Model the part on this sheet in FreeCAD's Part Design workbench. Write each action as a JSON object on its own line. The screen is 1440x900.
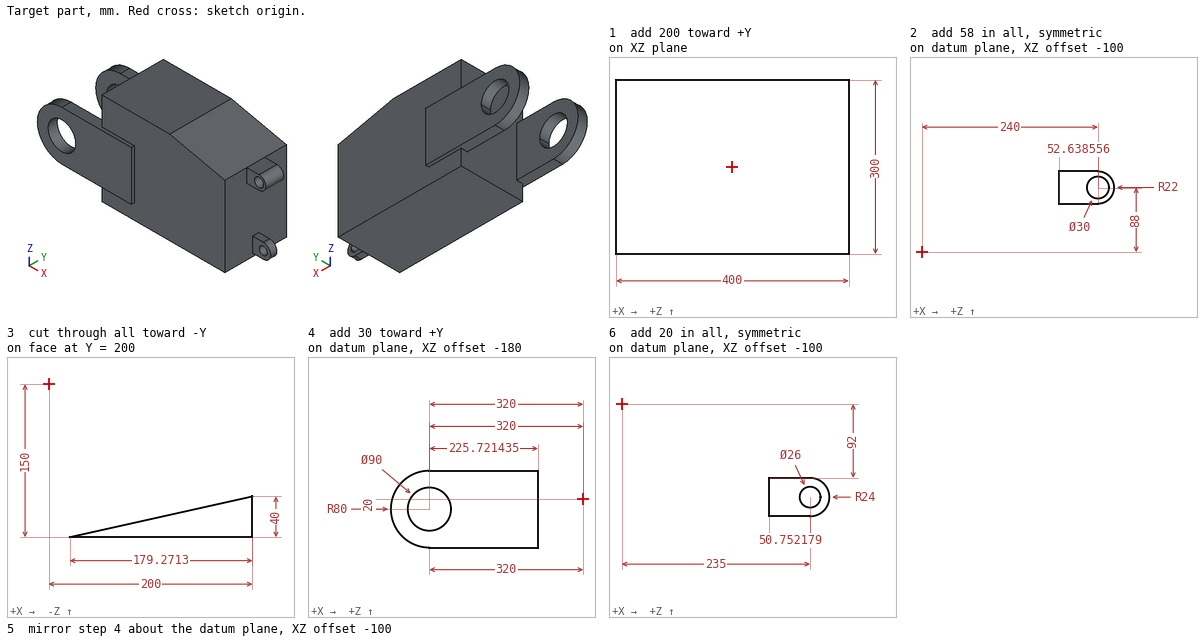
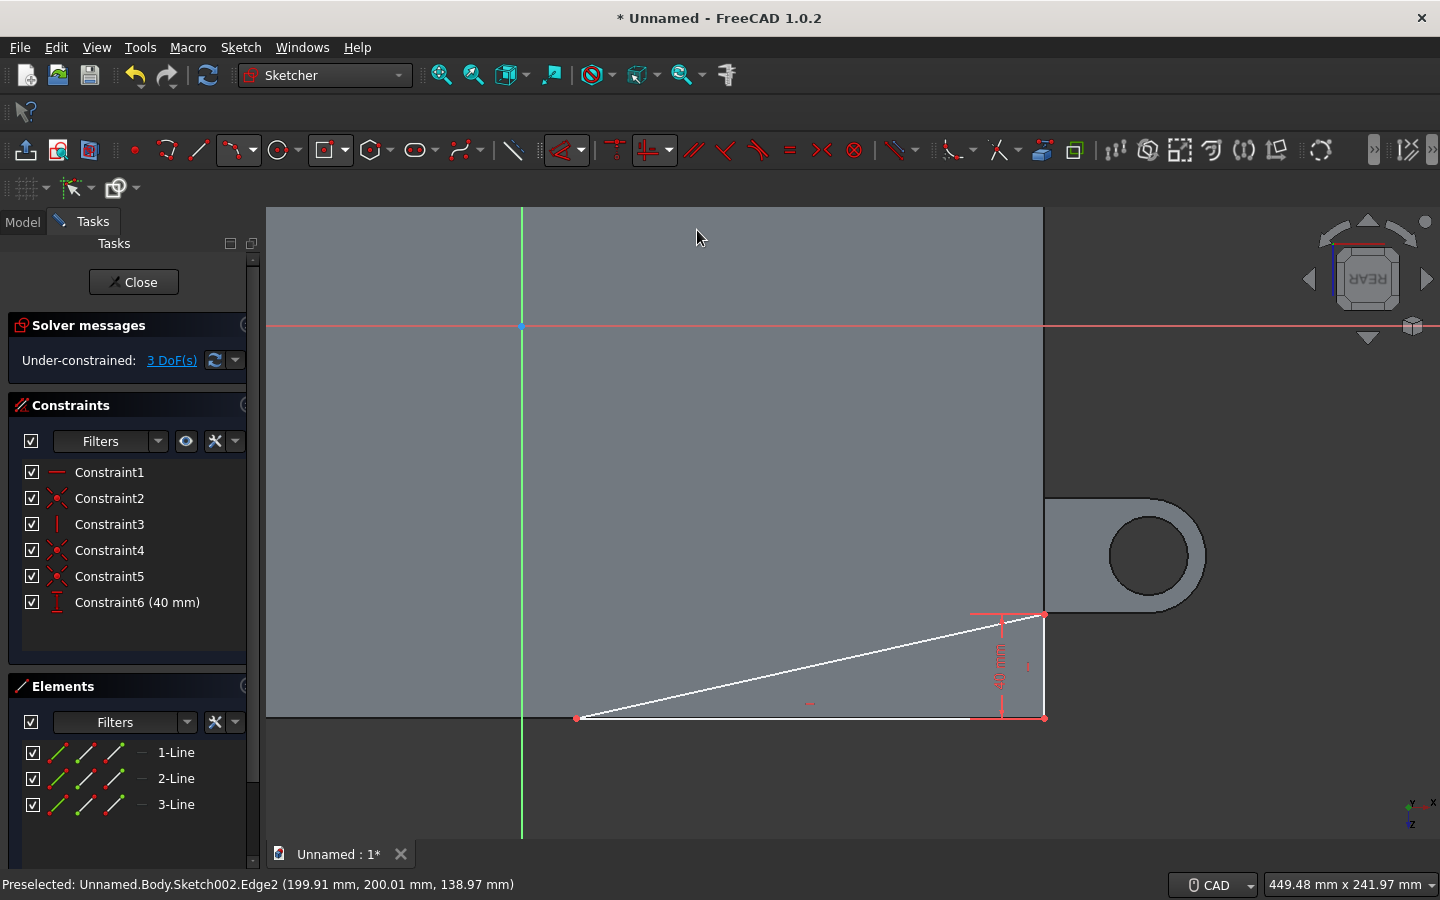
{"action": "left_click", "coordinate": [576, 719]}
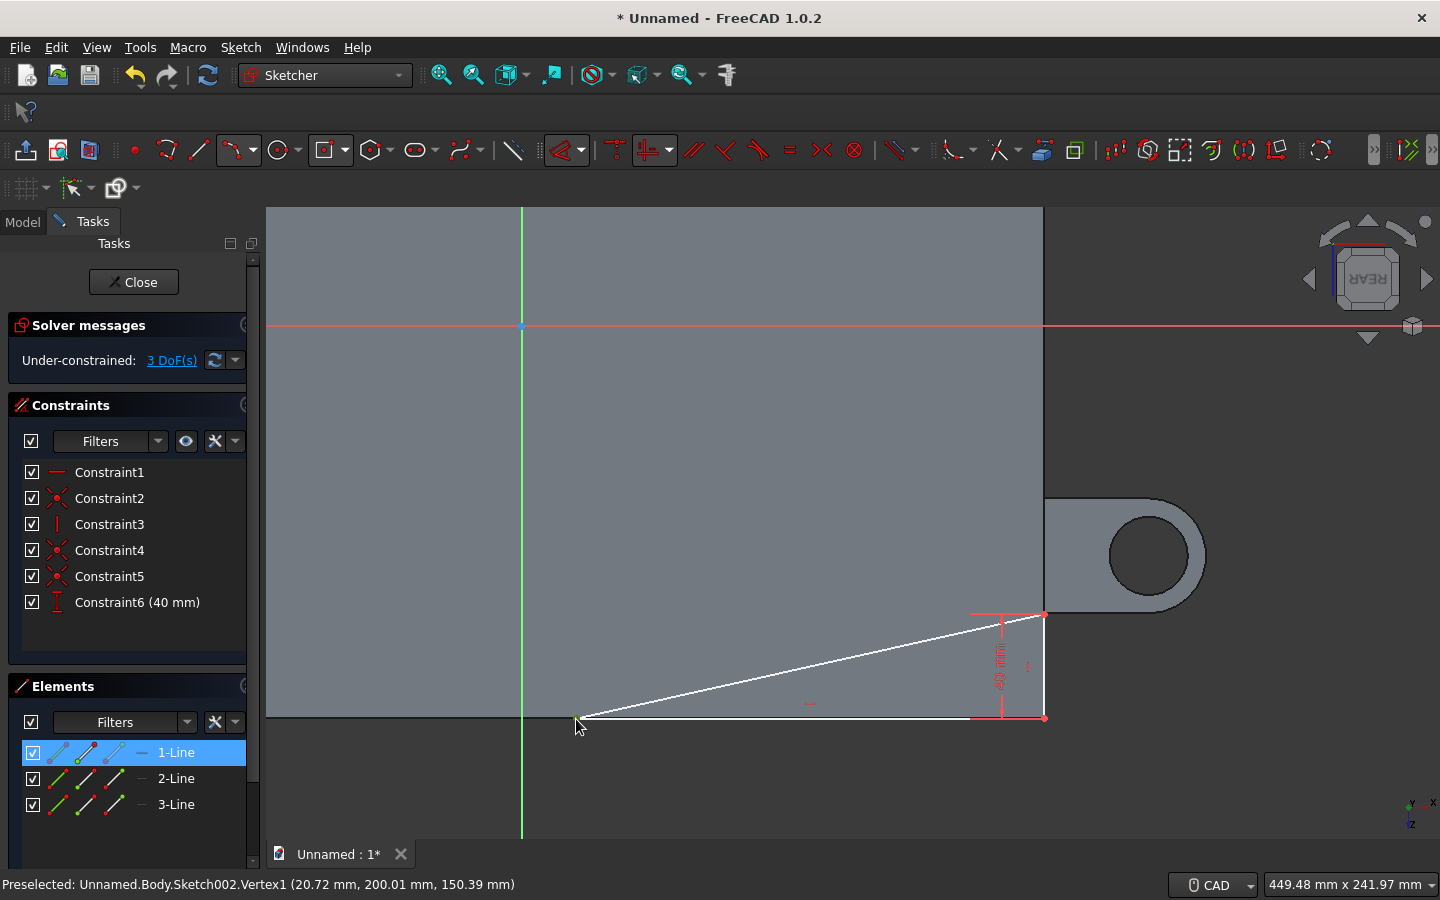
{"action": "left_click", "coordinate": [584, 150]}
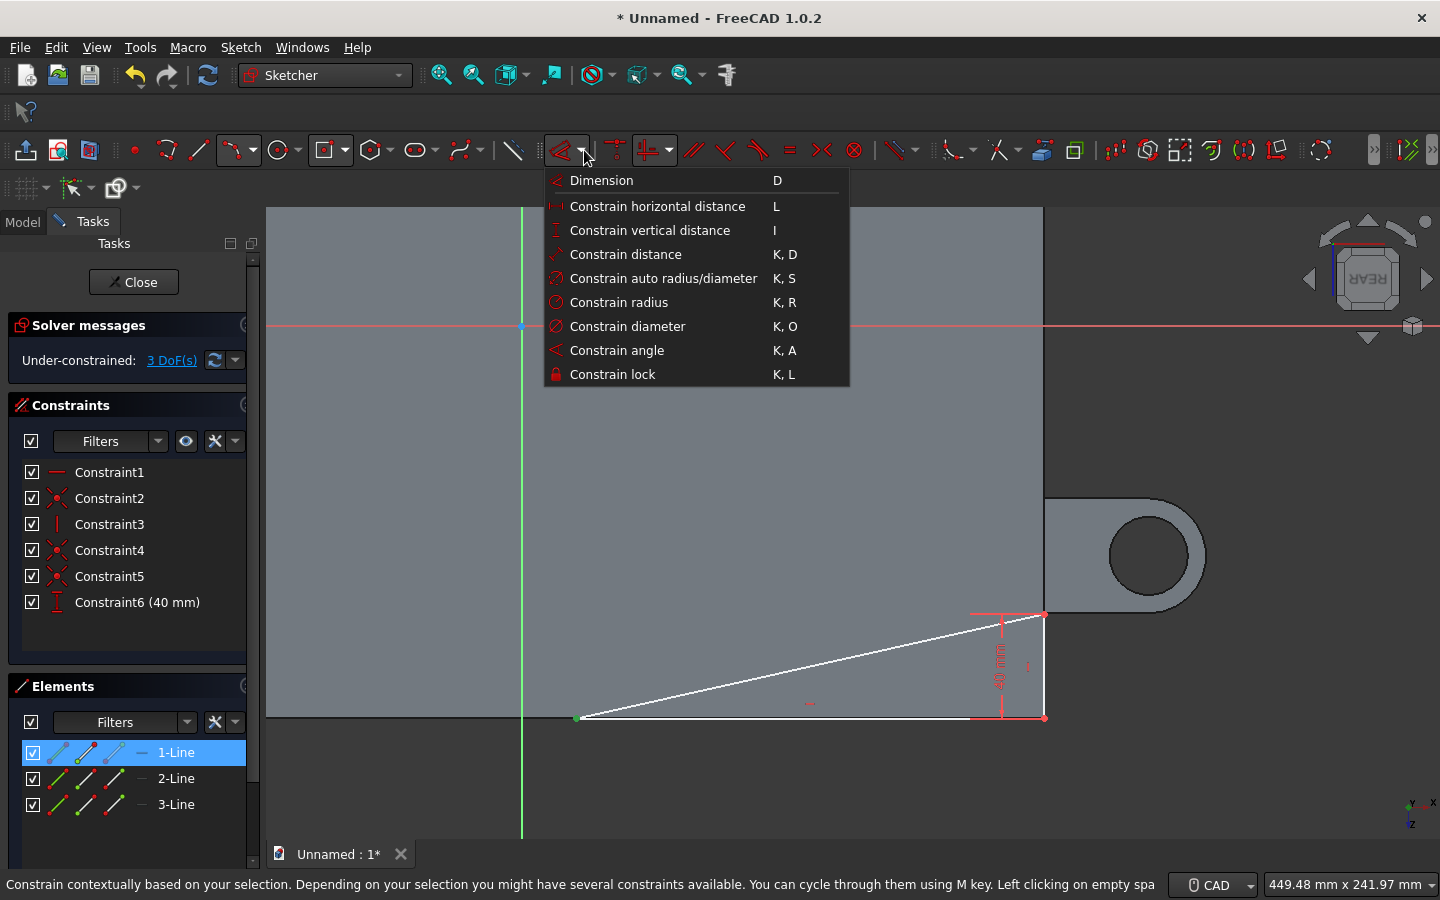
{"action": "left_click", "coordinate": [697, 230]}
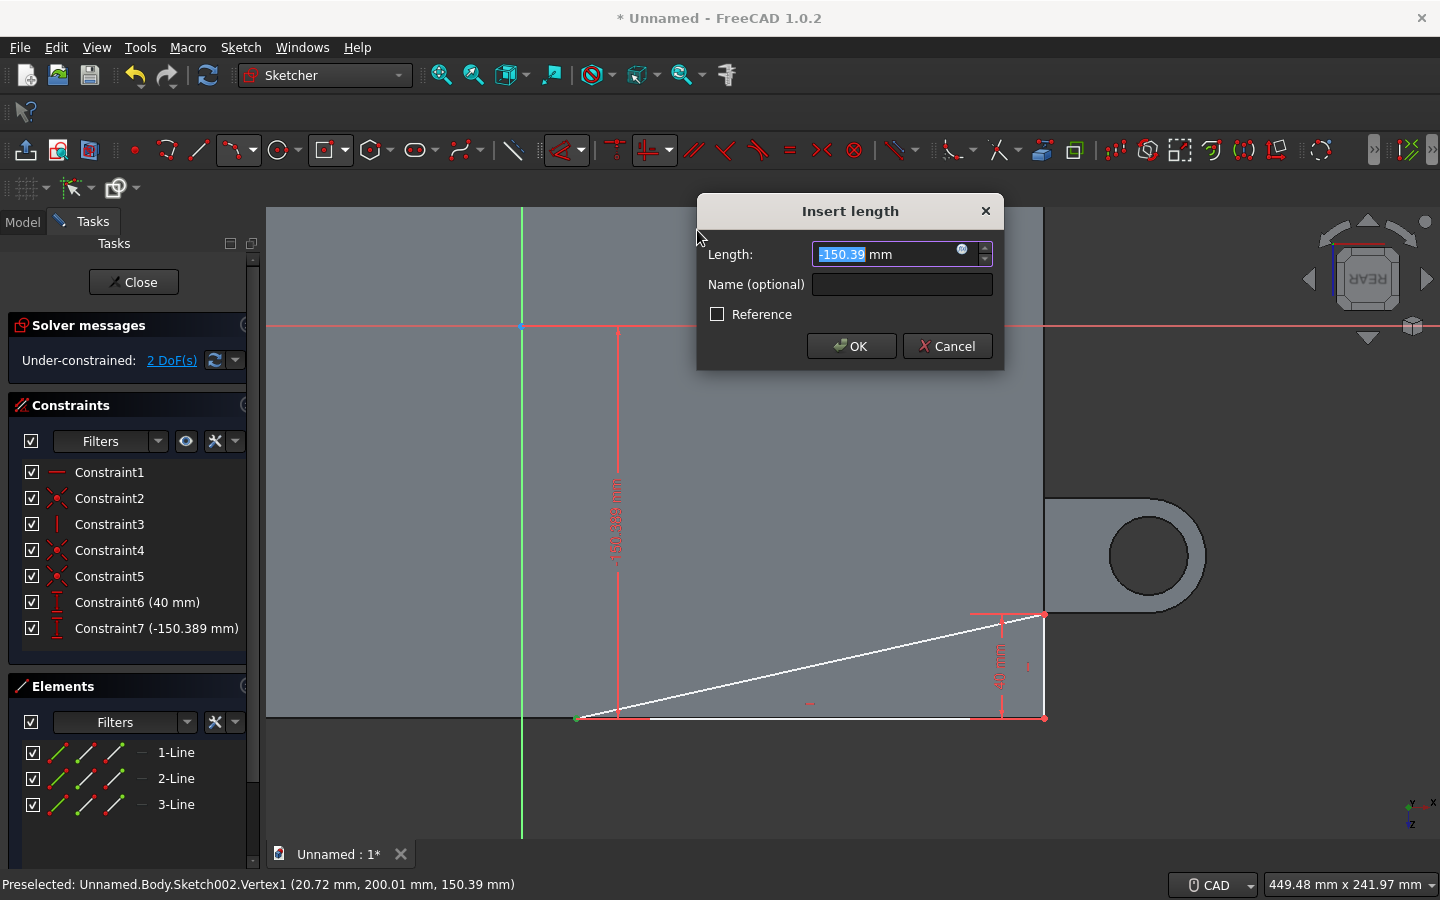
{"action": "type", "text": "-150"}
{"action": "key", "text": "Return"}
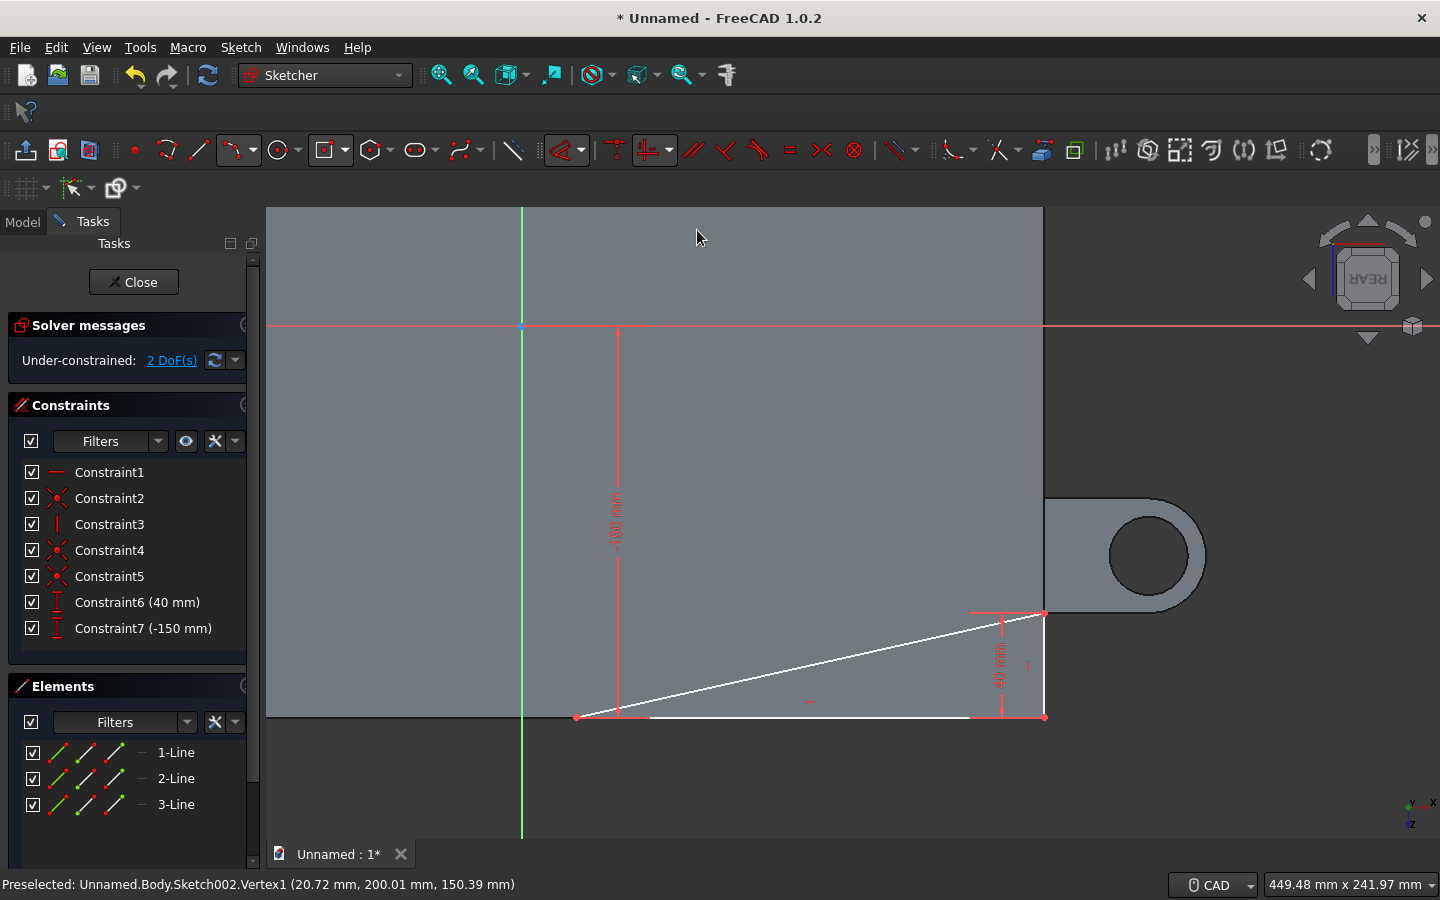
{"action": "left_click", "coordinate": [1044, 718]}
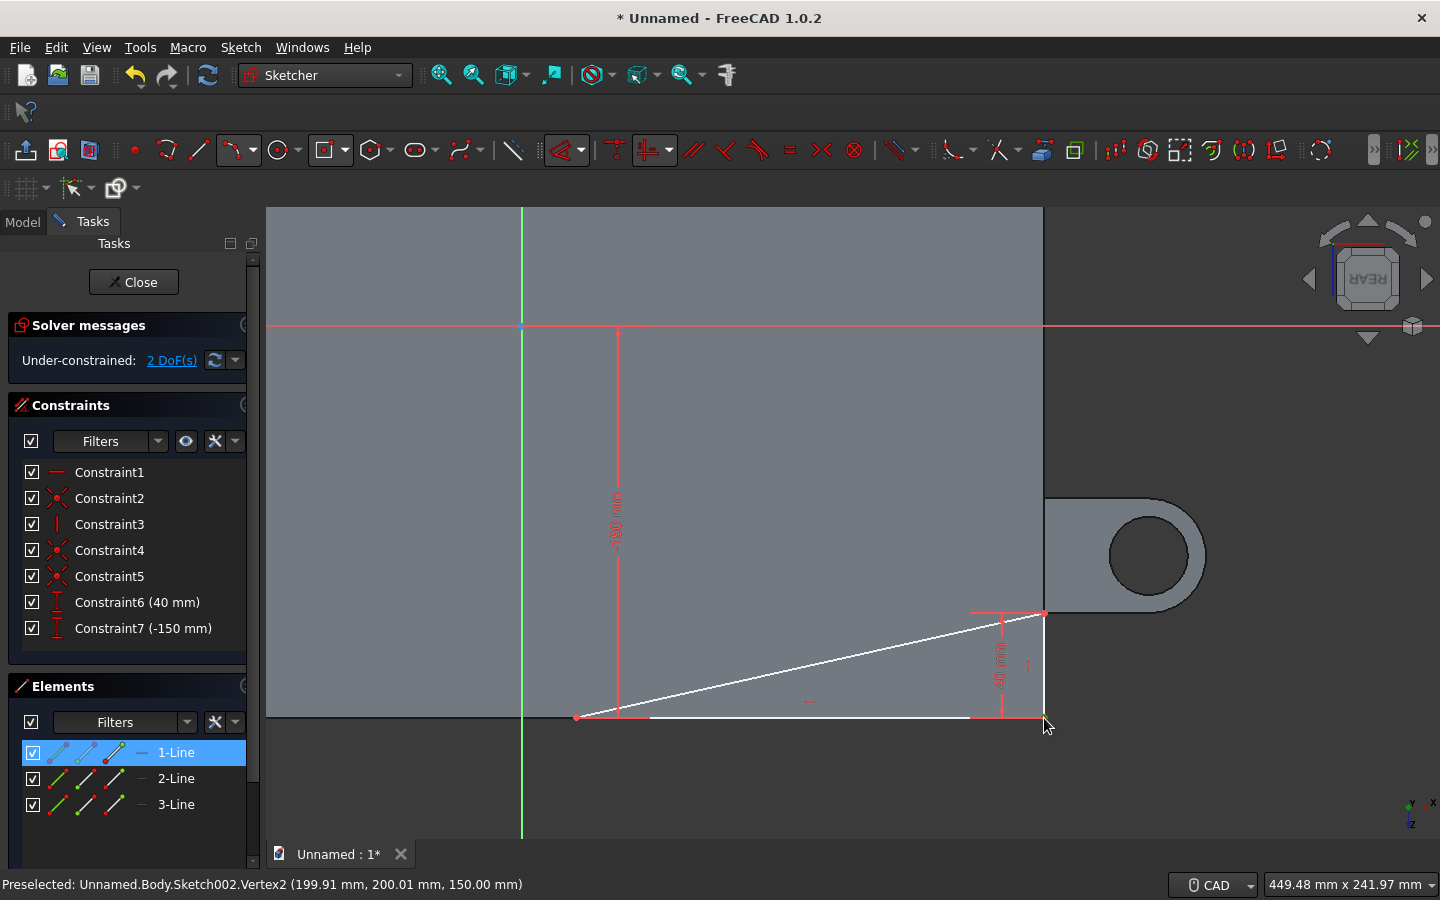
{"action": "left_click", "coordinate": [584, 150]}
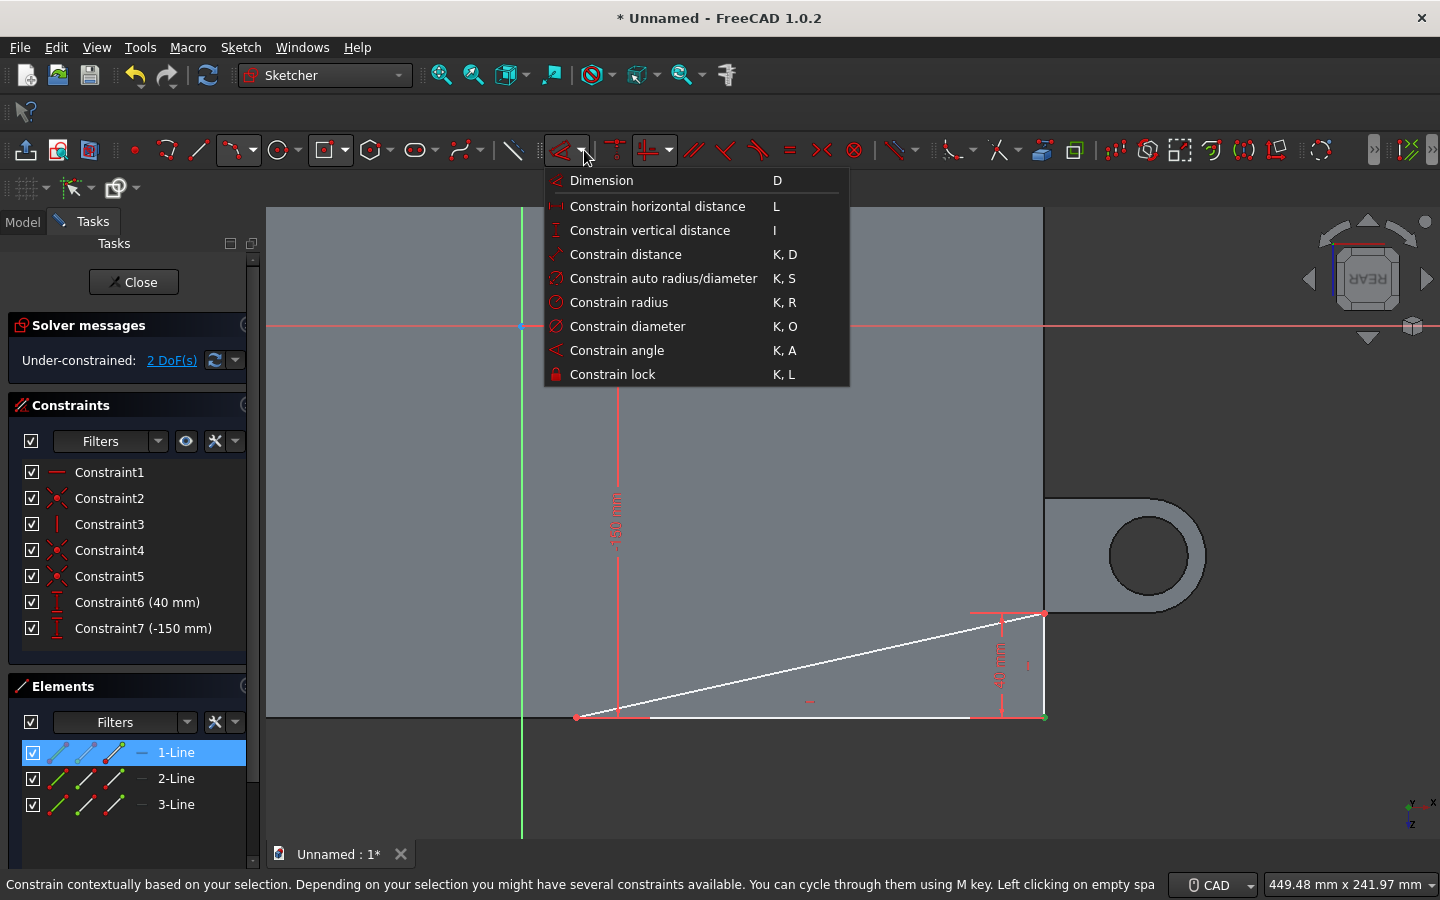
{"action": "left_click", "coordinate": [697, 206]}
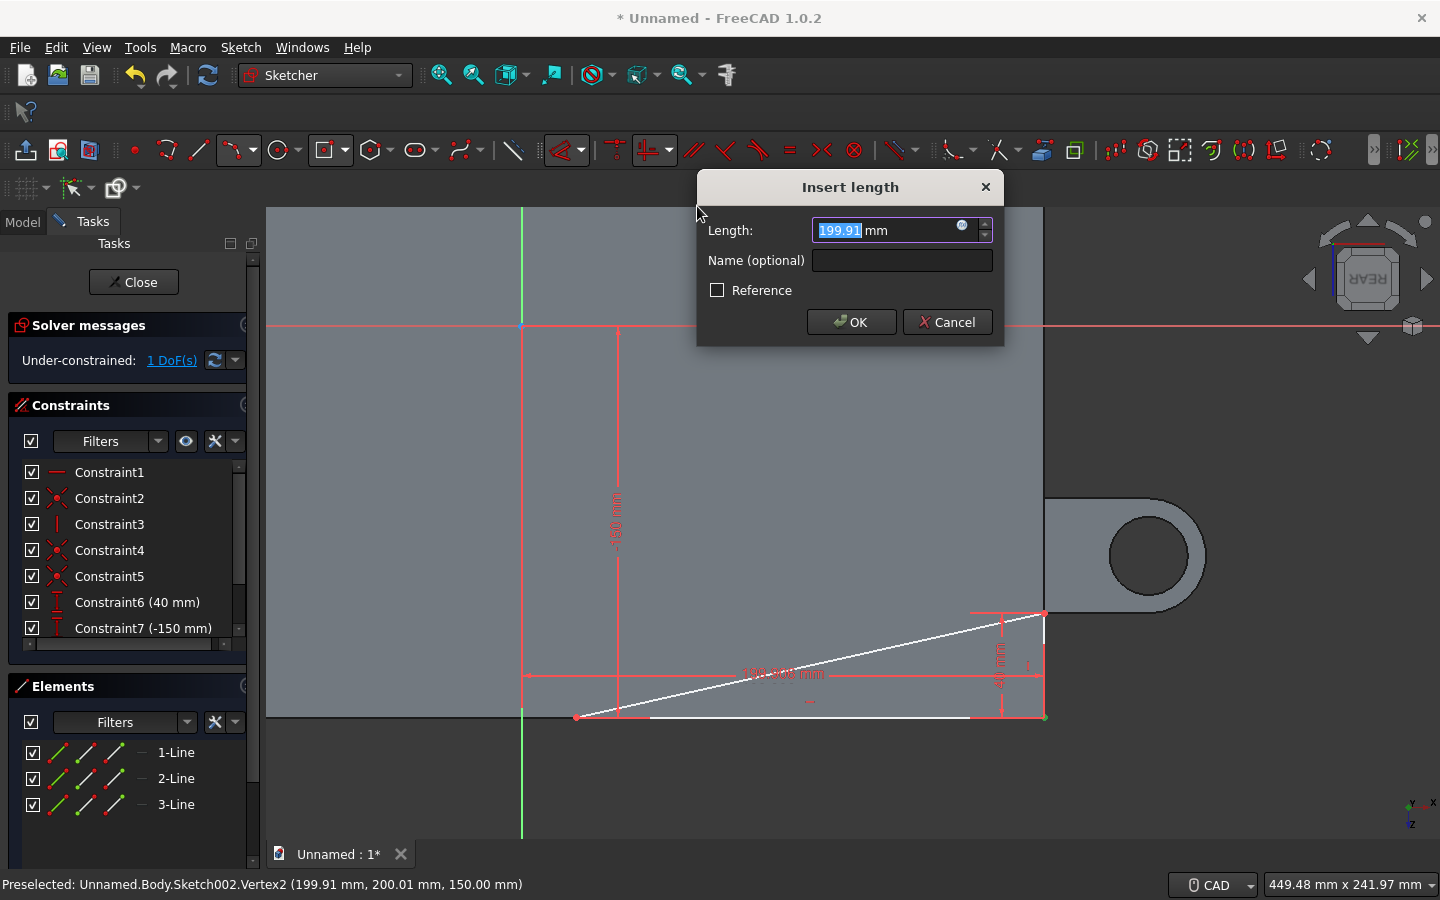
{"action": "type", "text": "200"}
{"action": "key", "text": "Return"}